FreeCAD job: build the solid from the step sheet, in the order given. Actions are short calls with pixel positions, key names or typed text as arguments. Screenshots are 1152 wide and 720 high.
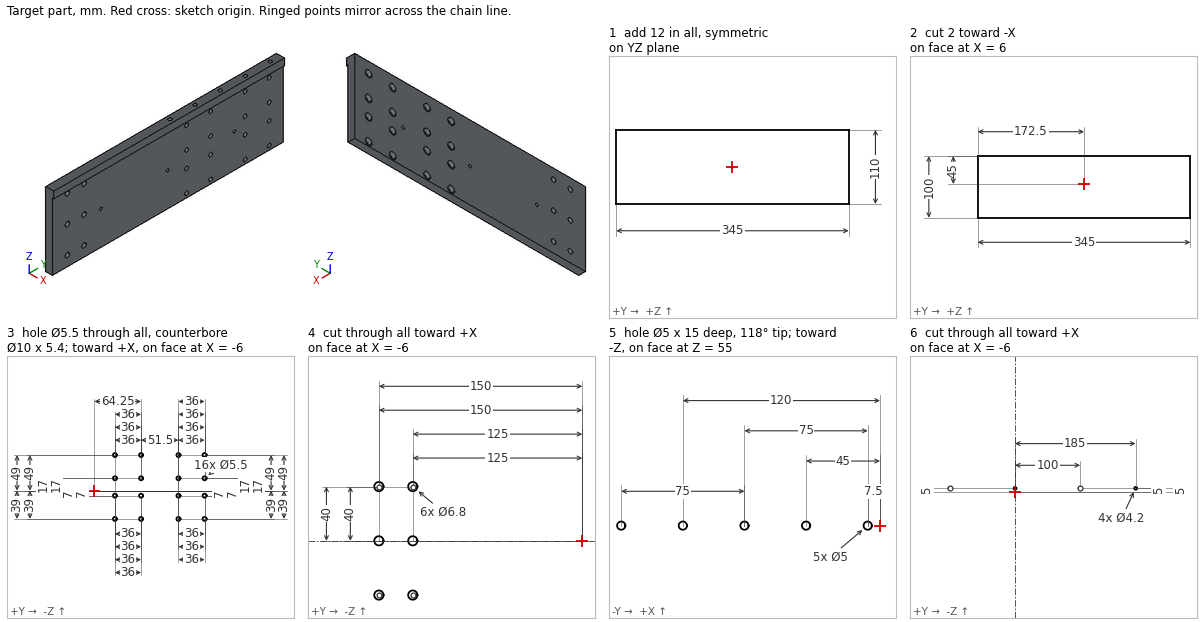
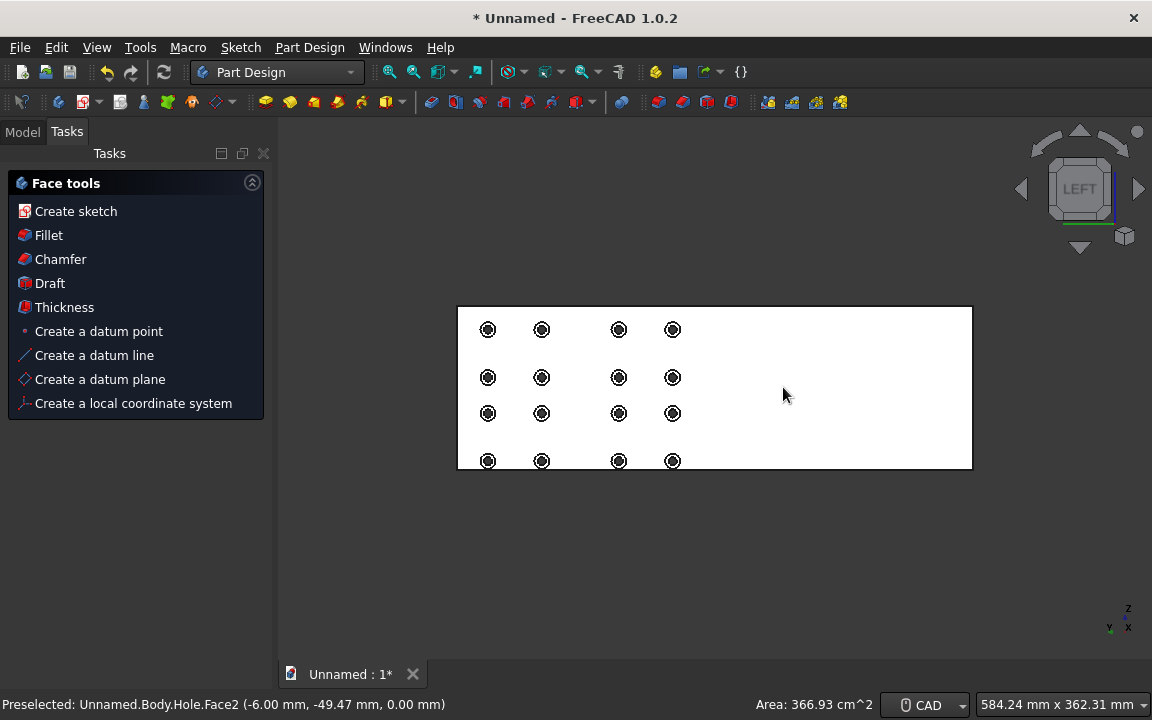
click(84, 102)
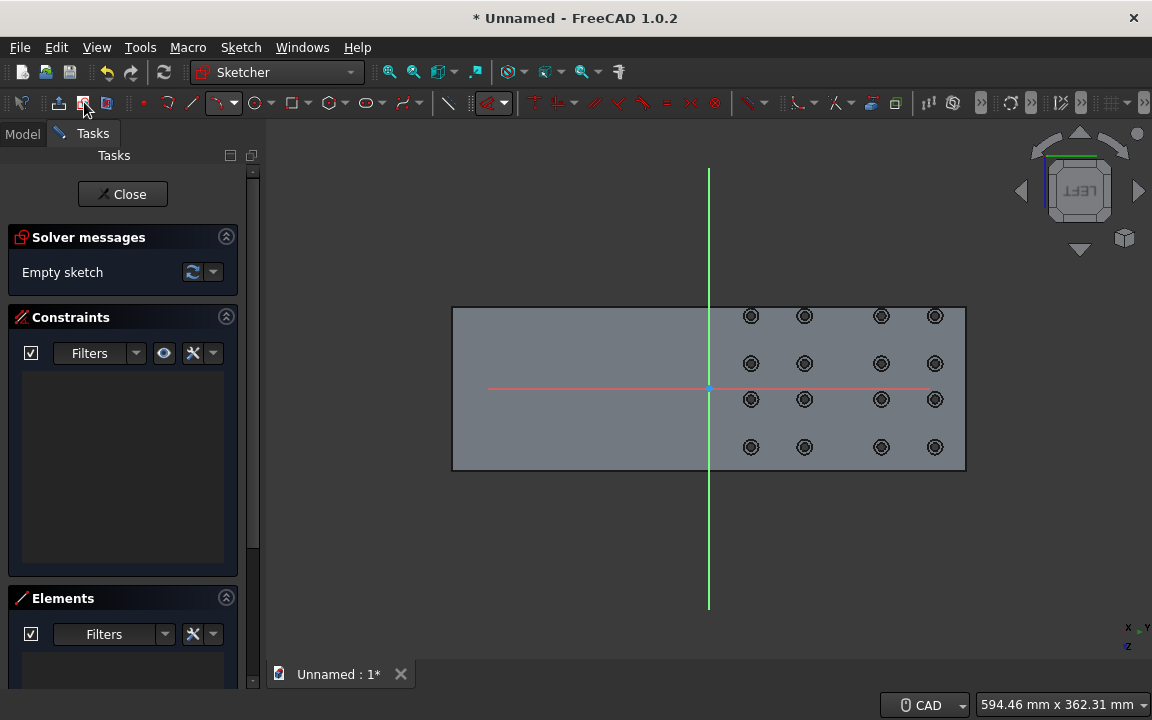
scroll(557, 389, up, 4)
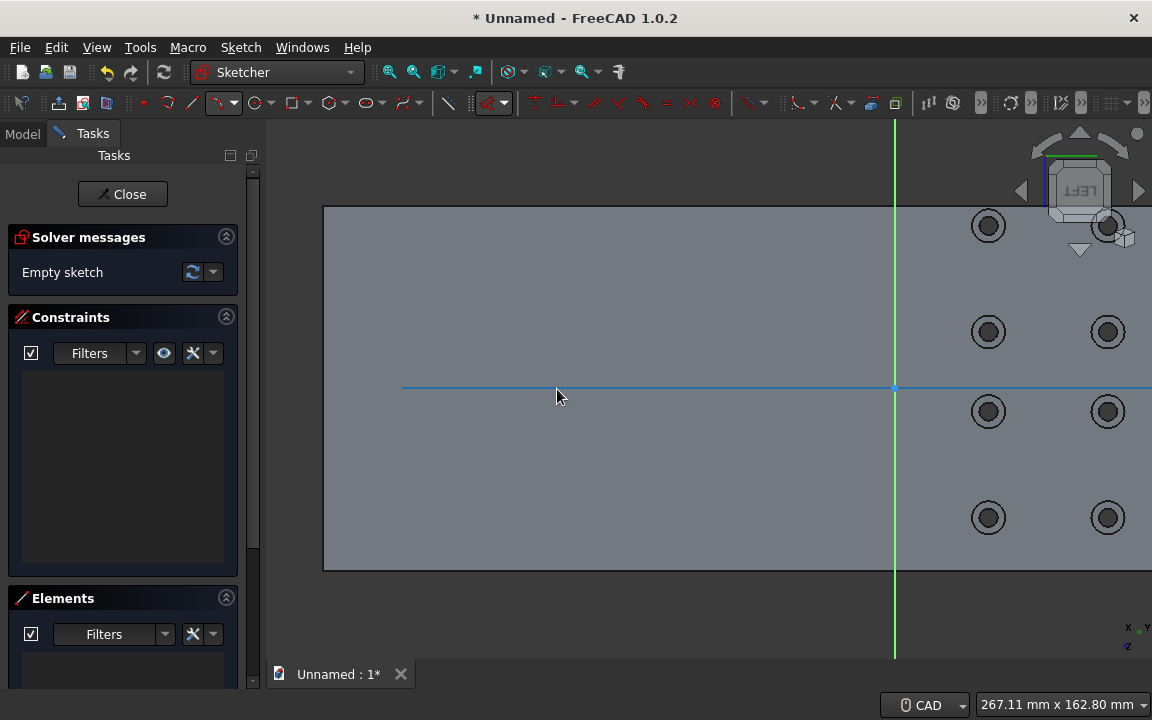
click(256, 104)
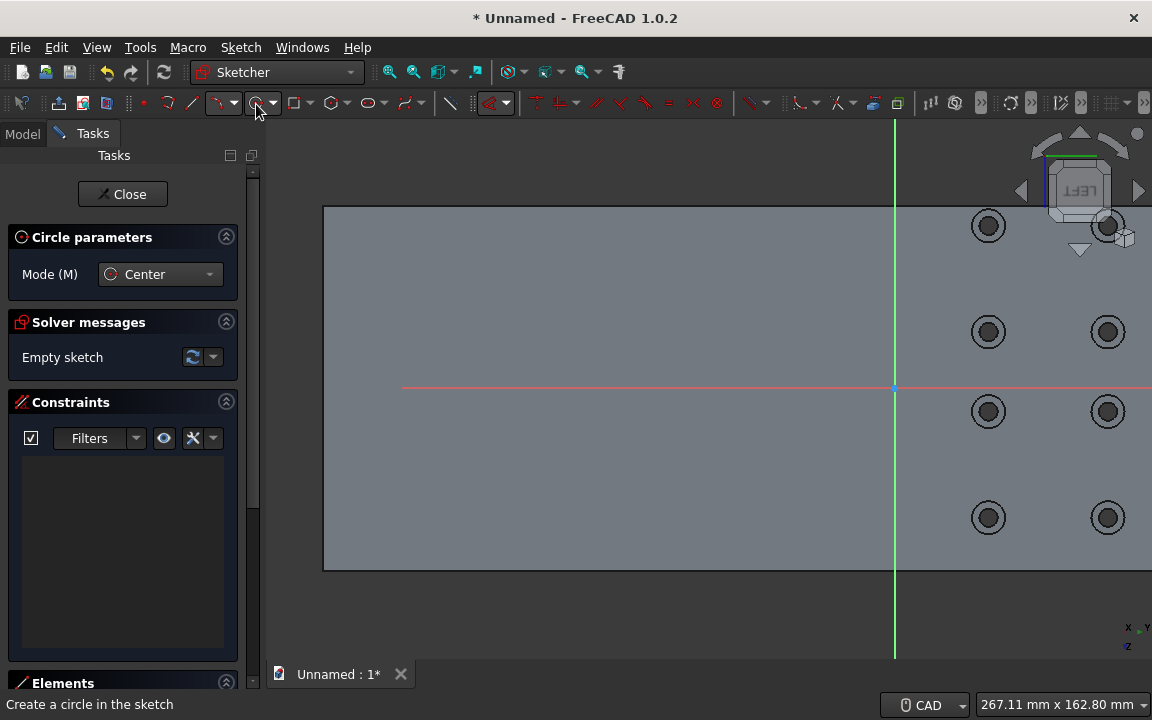
scroll(480, 256, up, 4)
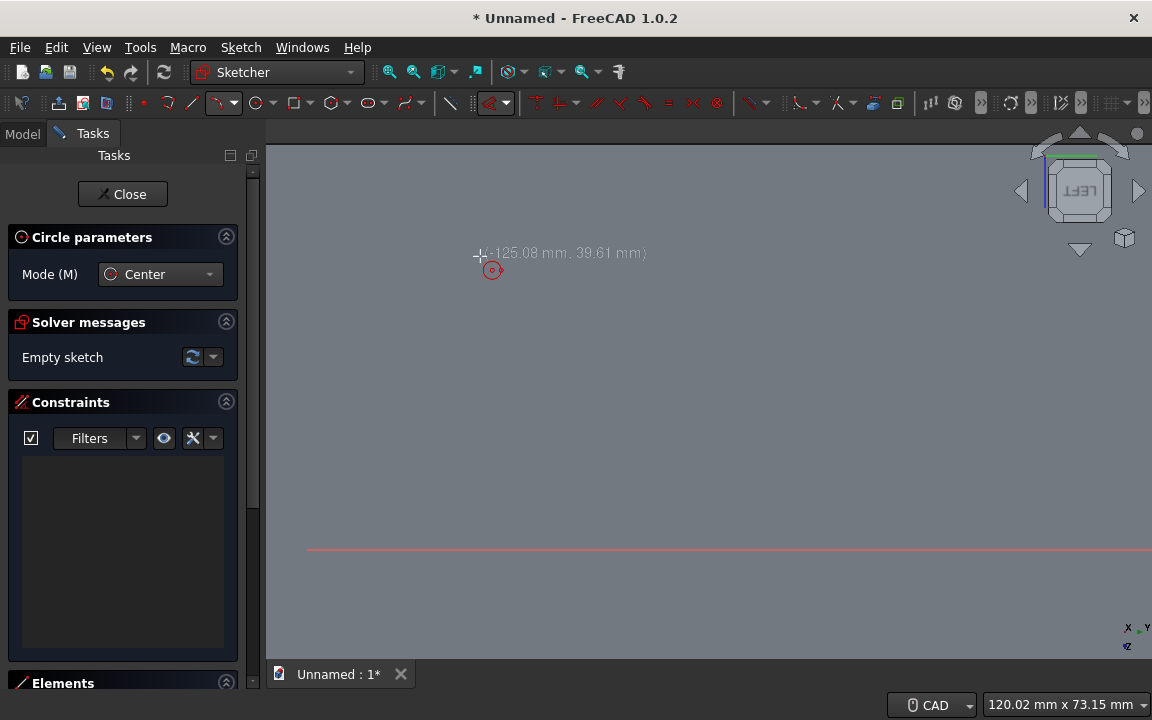
click(480, 255)
click(498, 237)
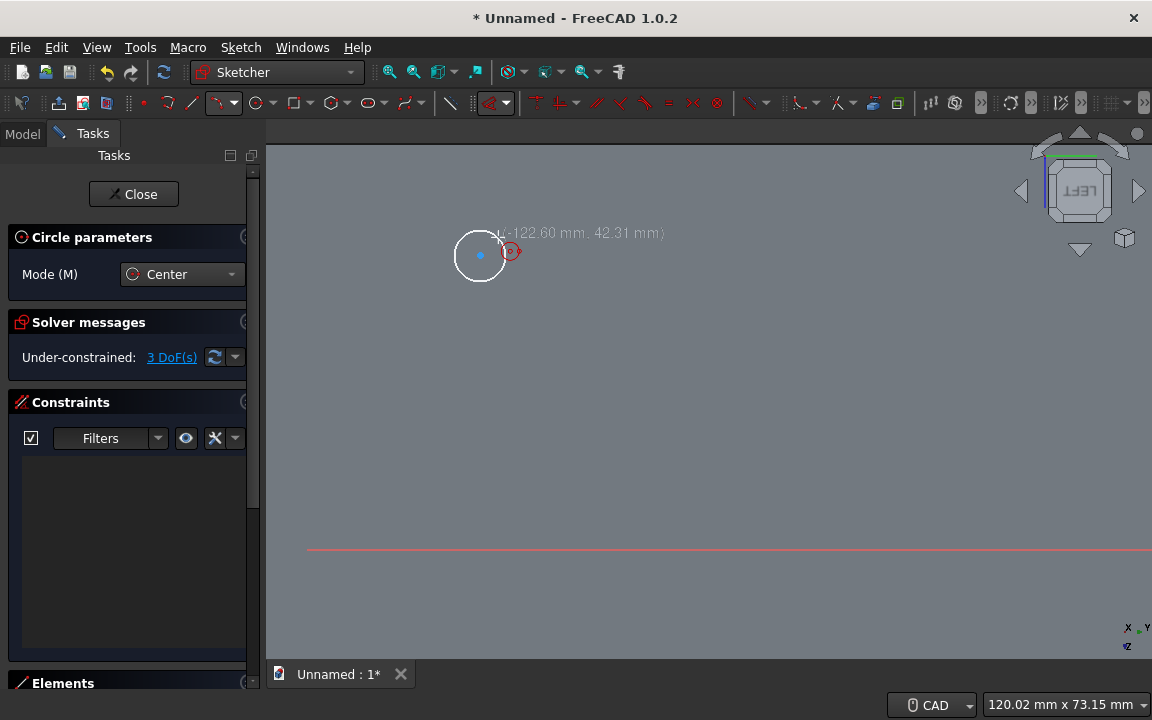
click(296, 255)
click(313, 237)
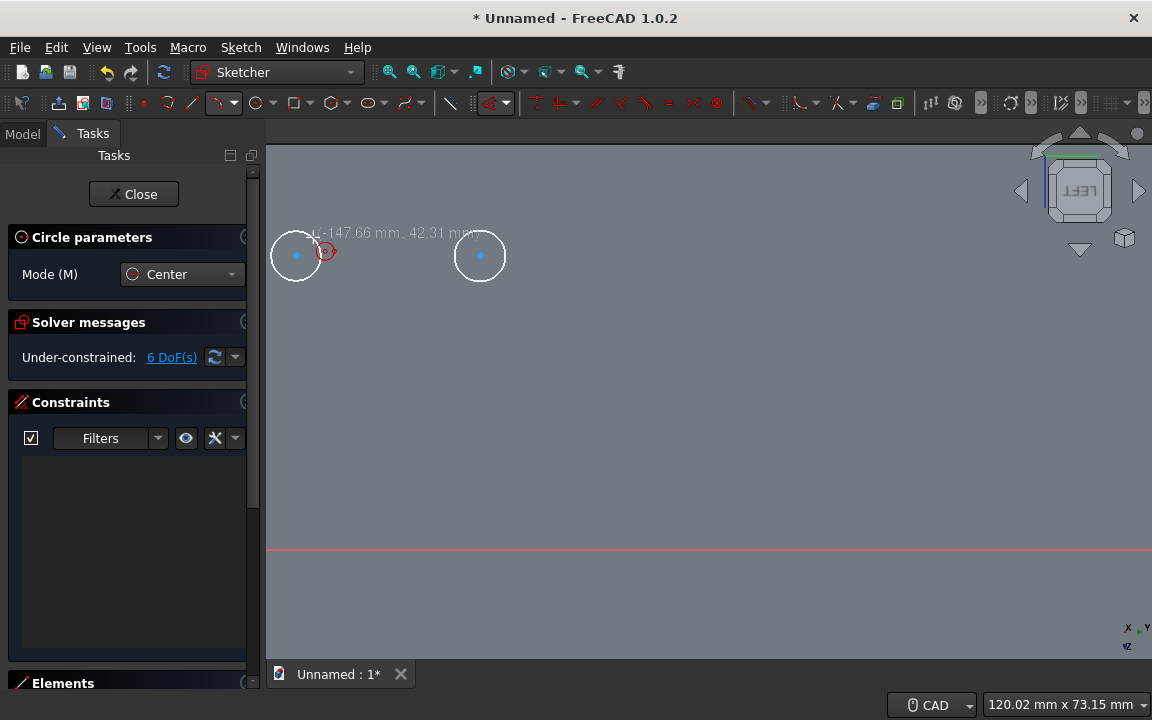
click(480, 550)
click(498, 533)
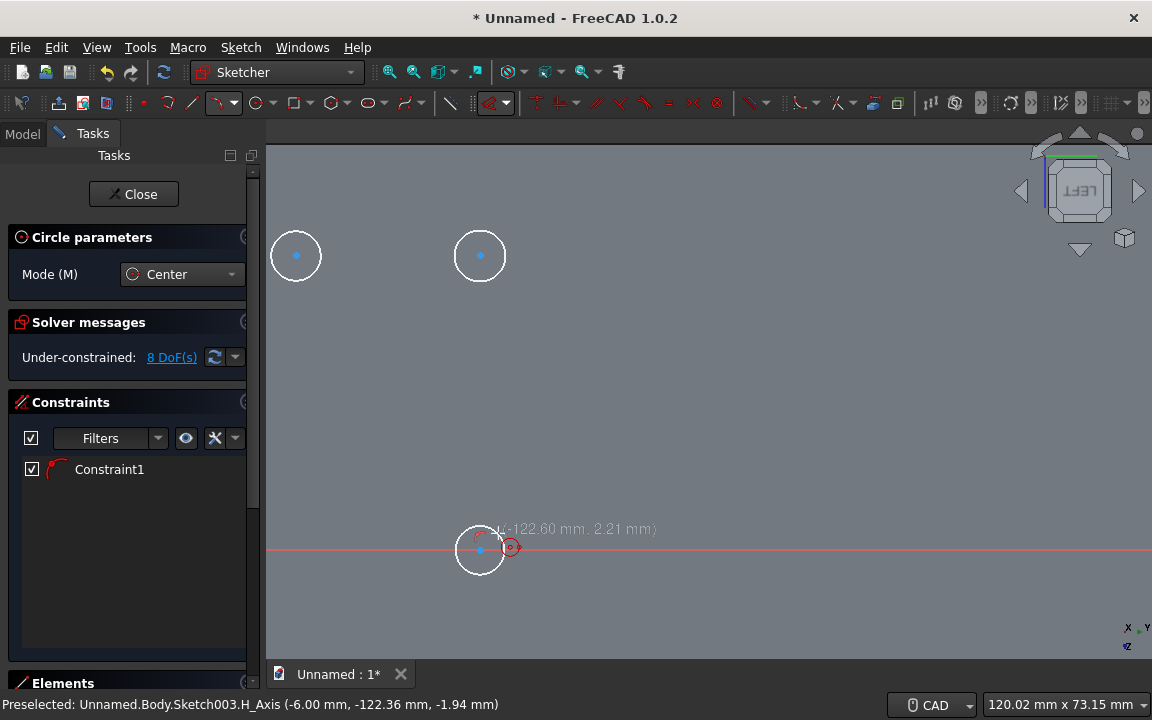
click(296, 550)
click(313, 533)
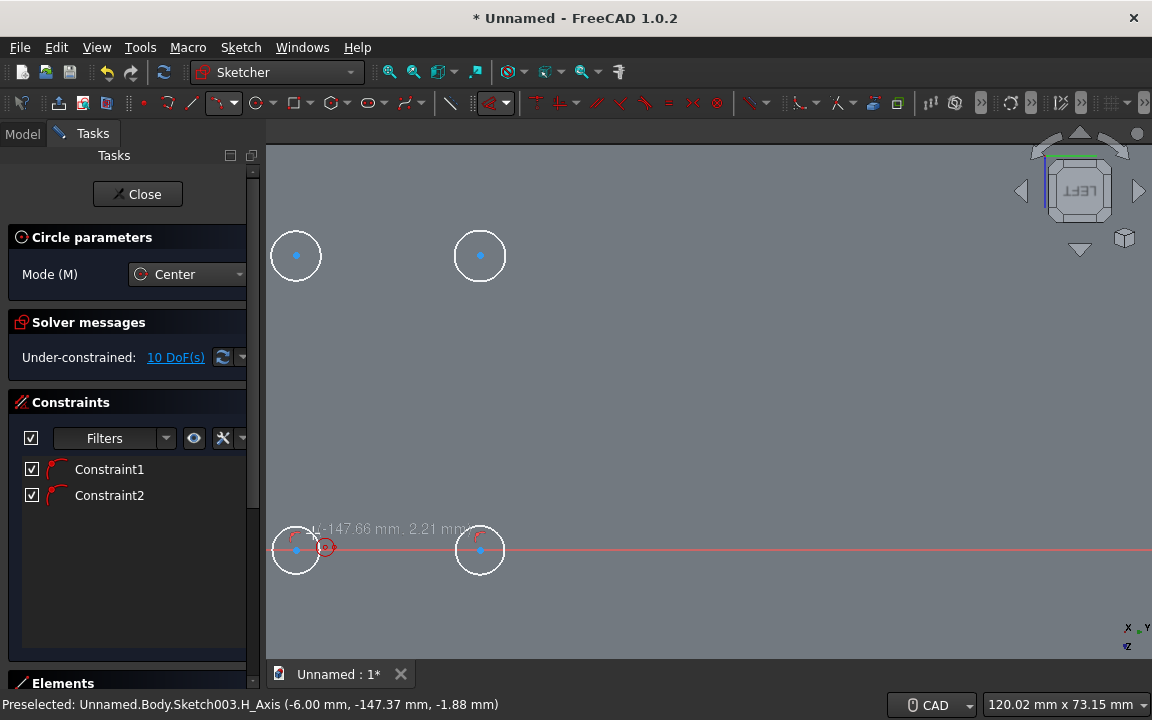
scroll(480, 257, down, 4)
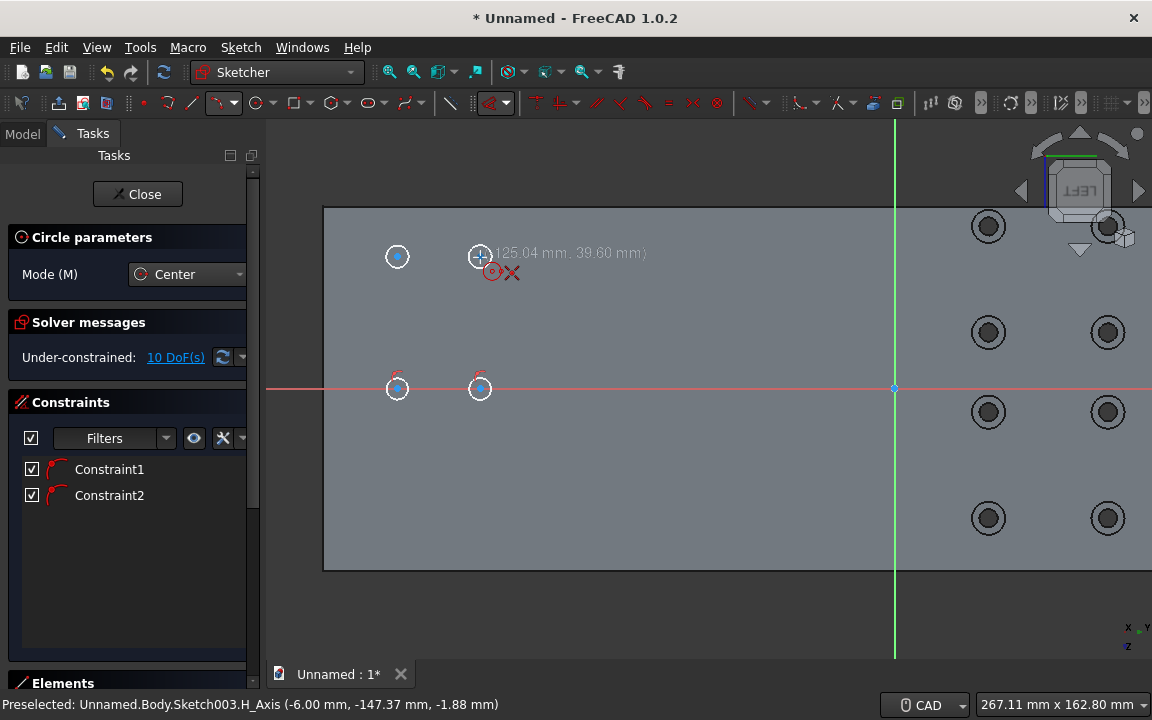
scroll(480, 522, up, 4)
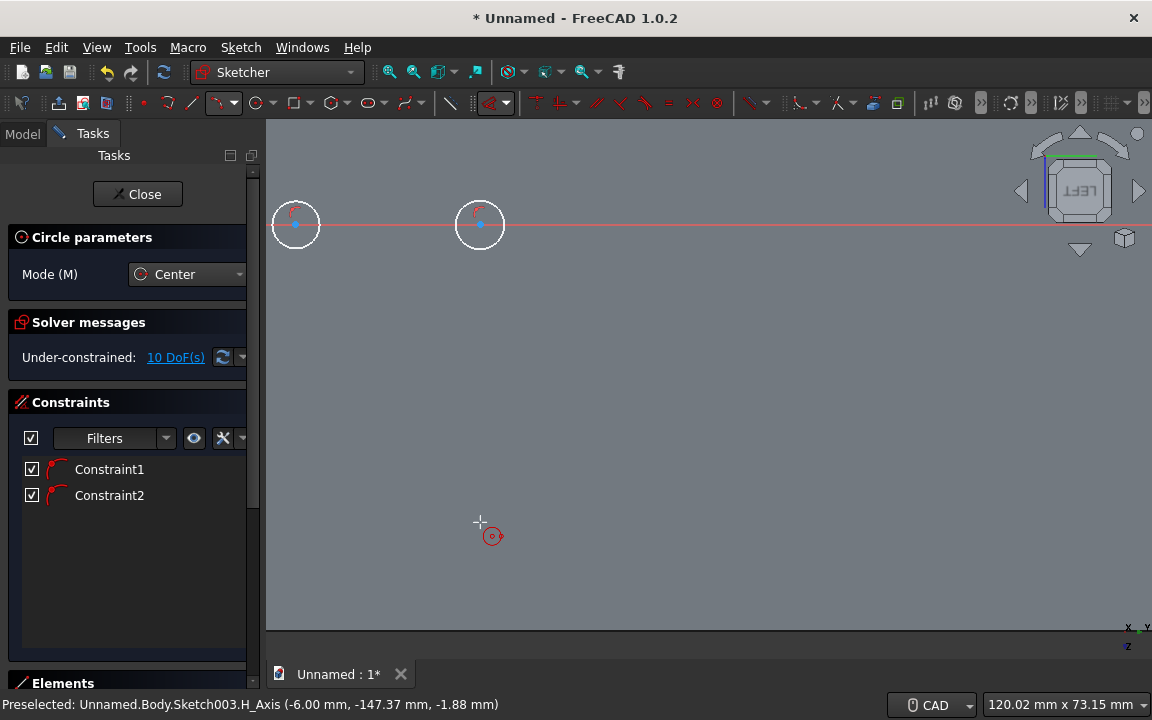
click(480, 520)
click(498, 502)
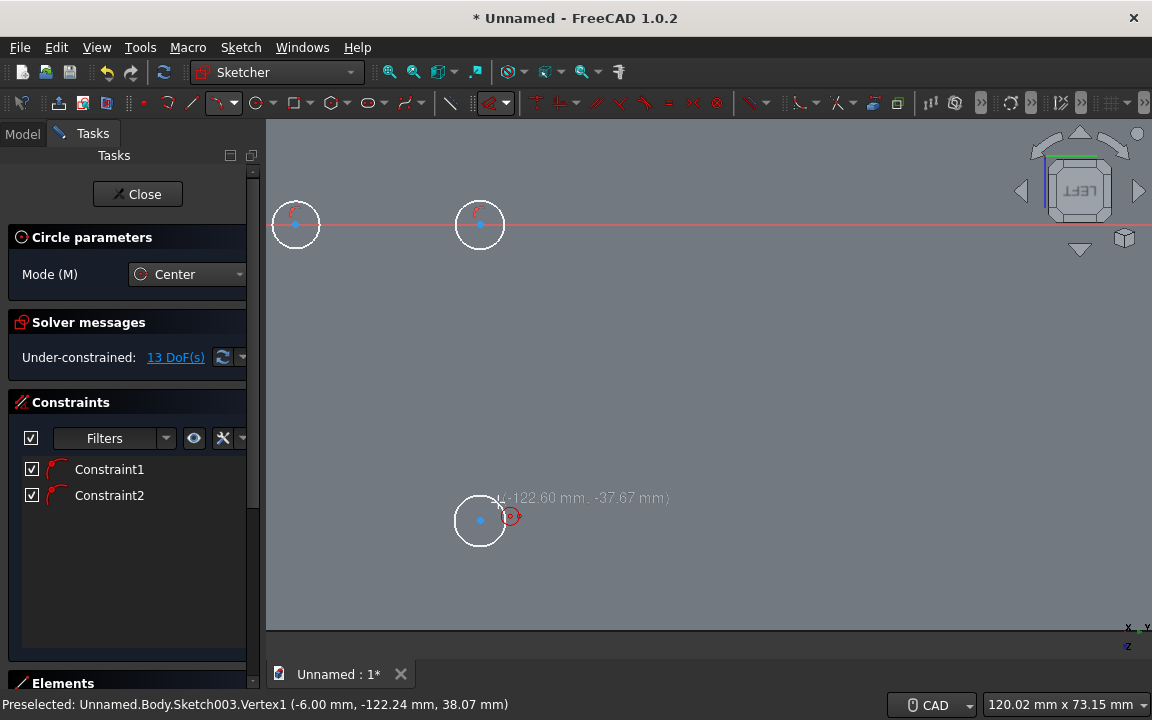
click(296, 520)
click(313, 502)
key(Escape)